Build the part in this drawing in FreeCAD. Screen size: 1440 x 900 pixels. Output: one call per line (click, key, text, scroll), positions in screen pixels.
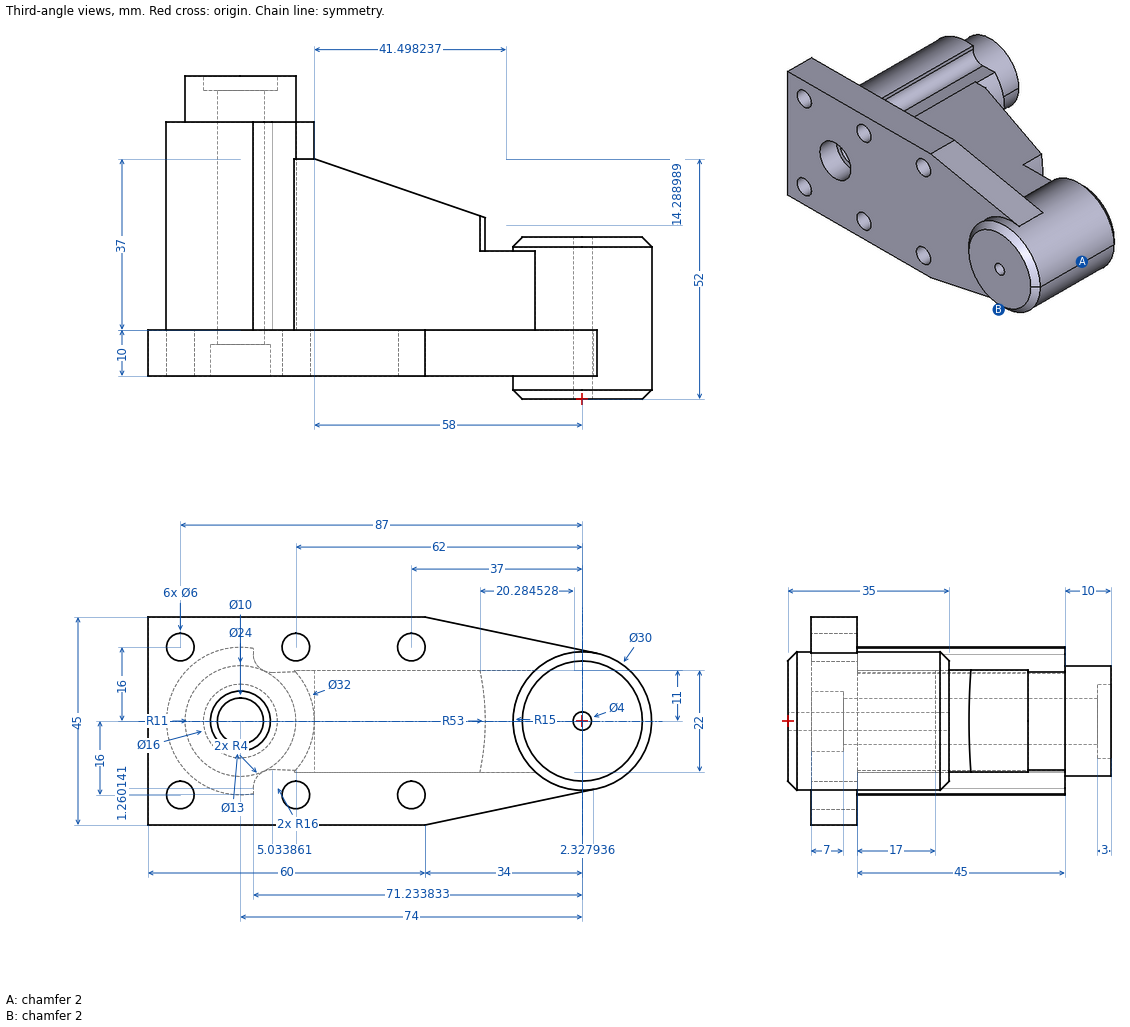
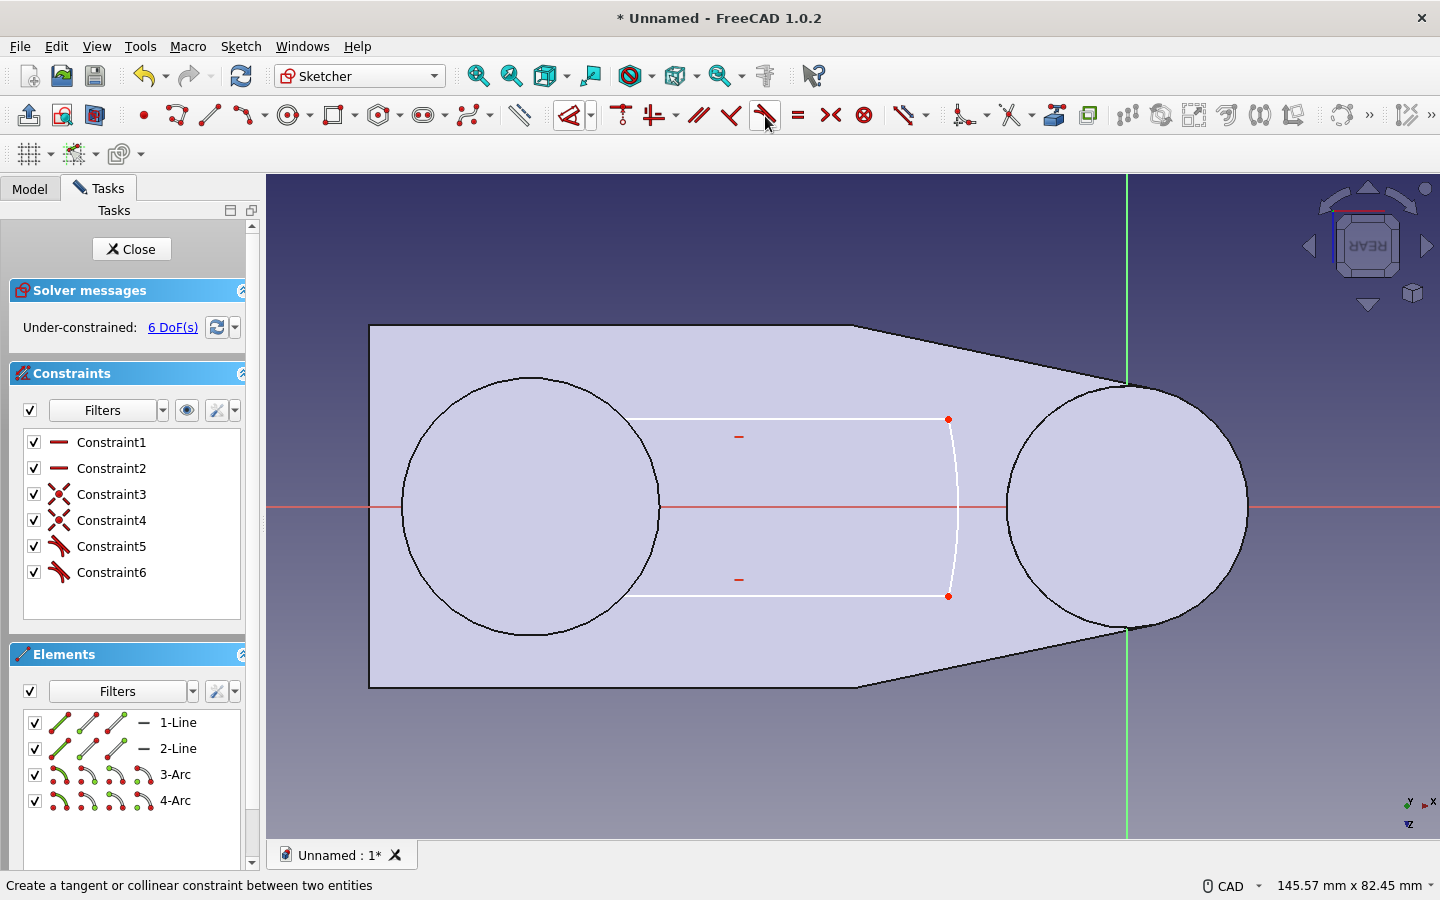
click(459, 456)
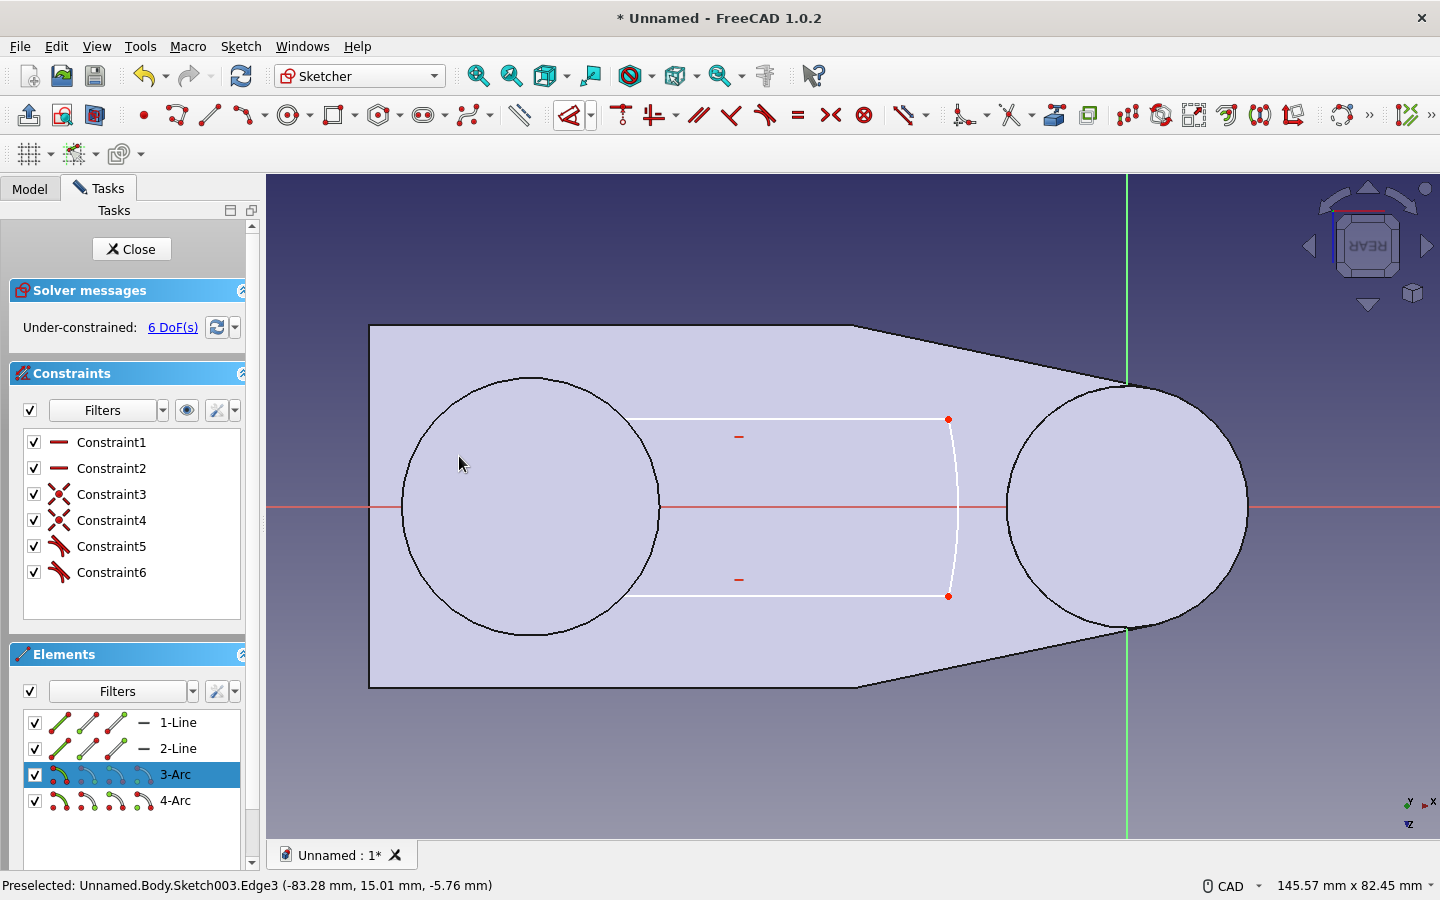
click(957, 544)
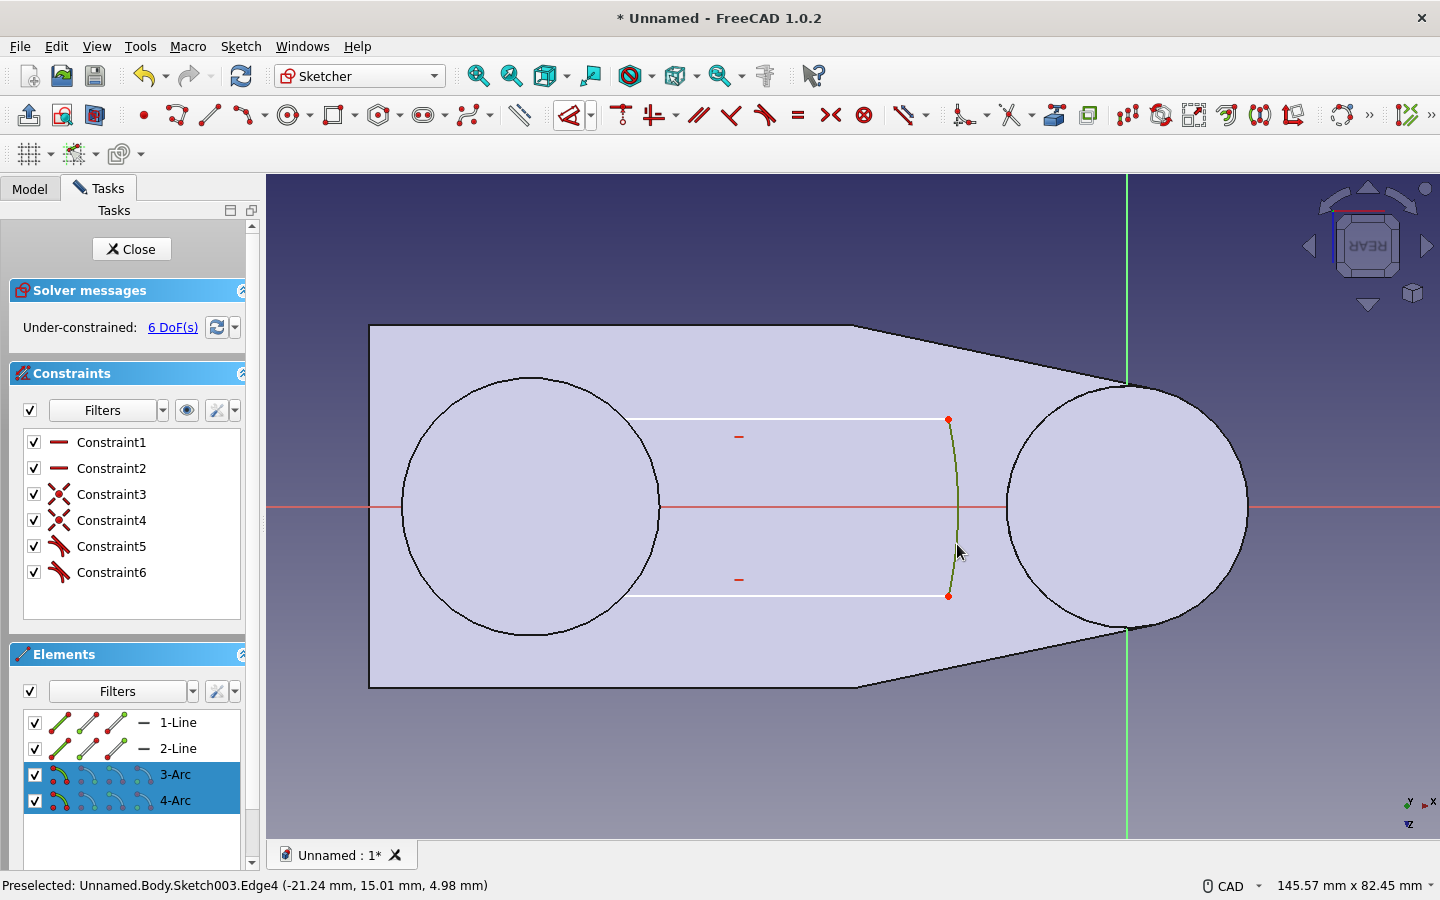
click(621, 116)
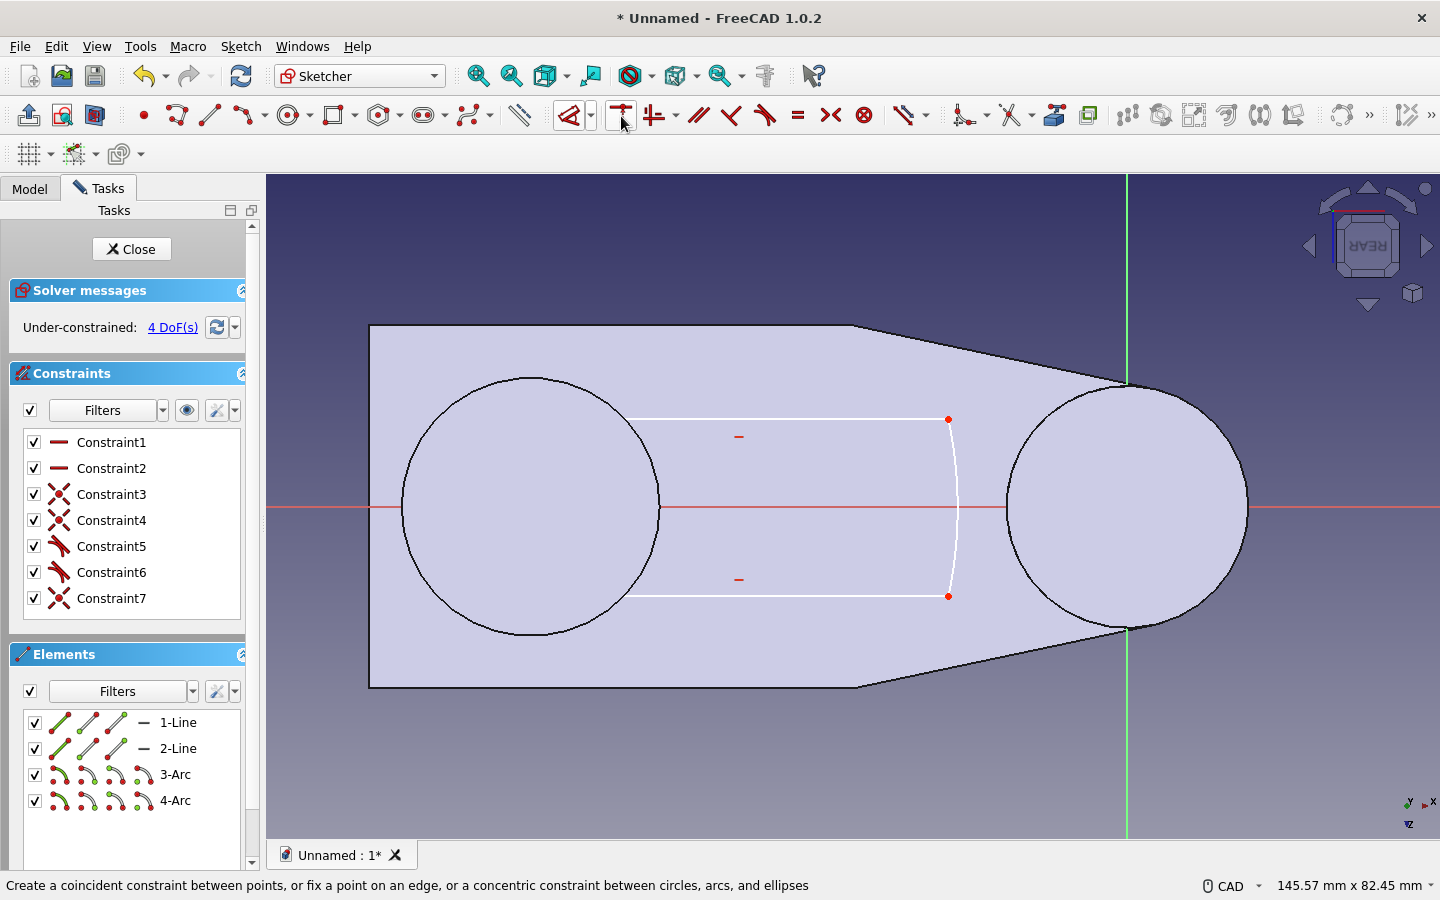
click(531, 508)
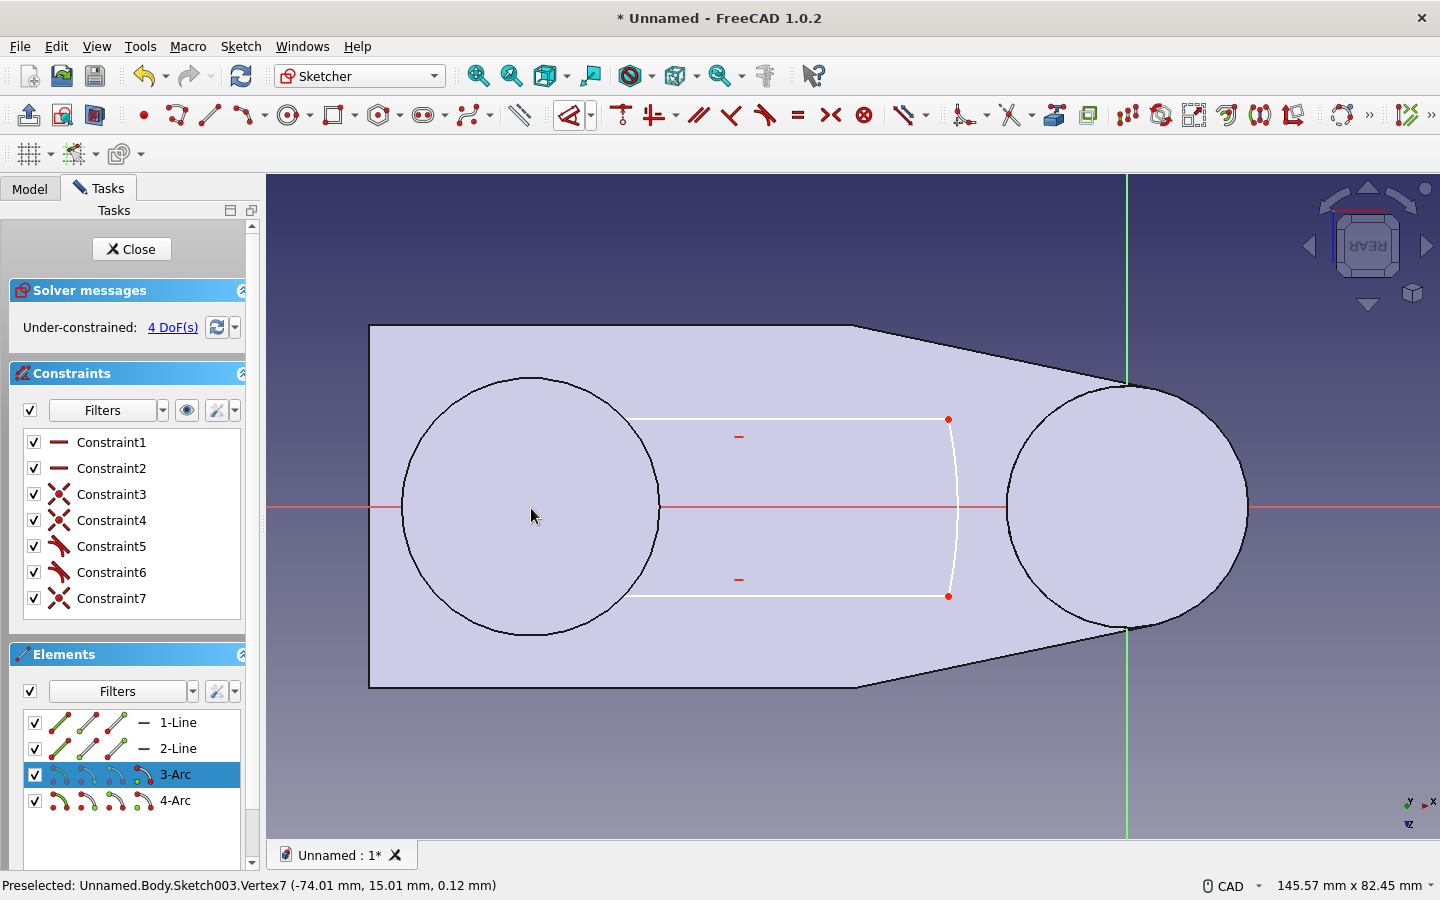
click(364, 507)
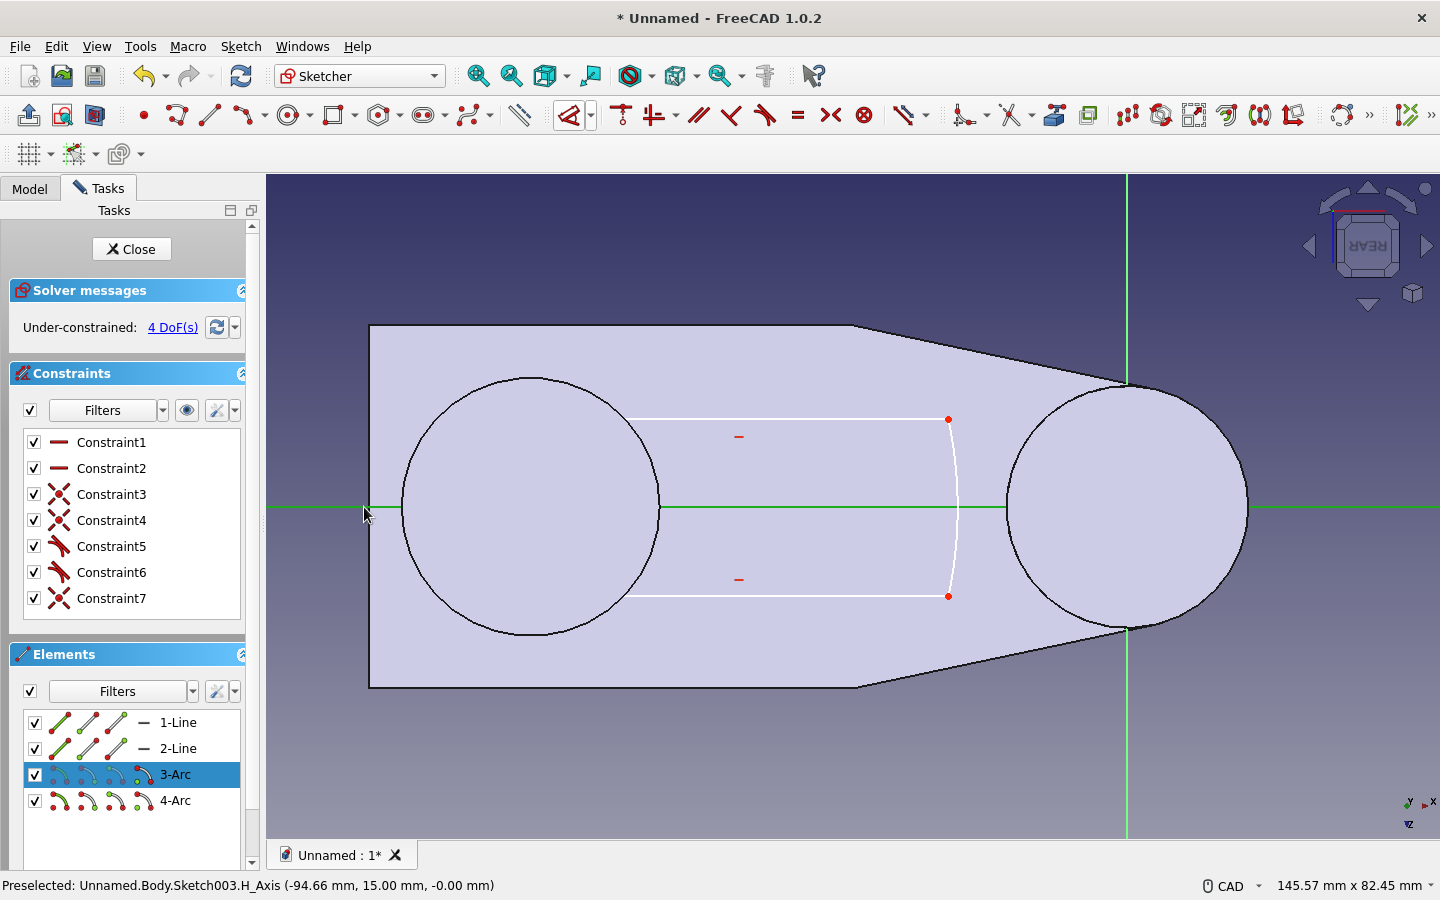
click(621, 116)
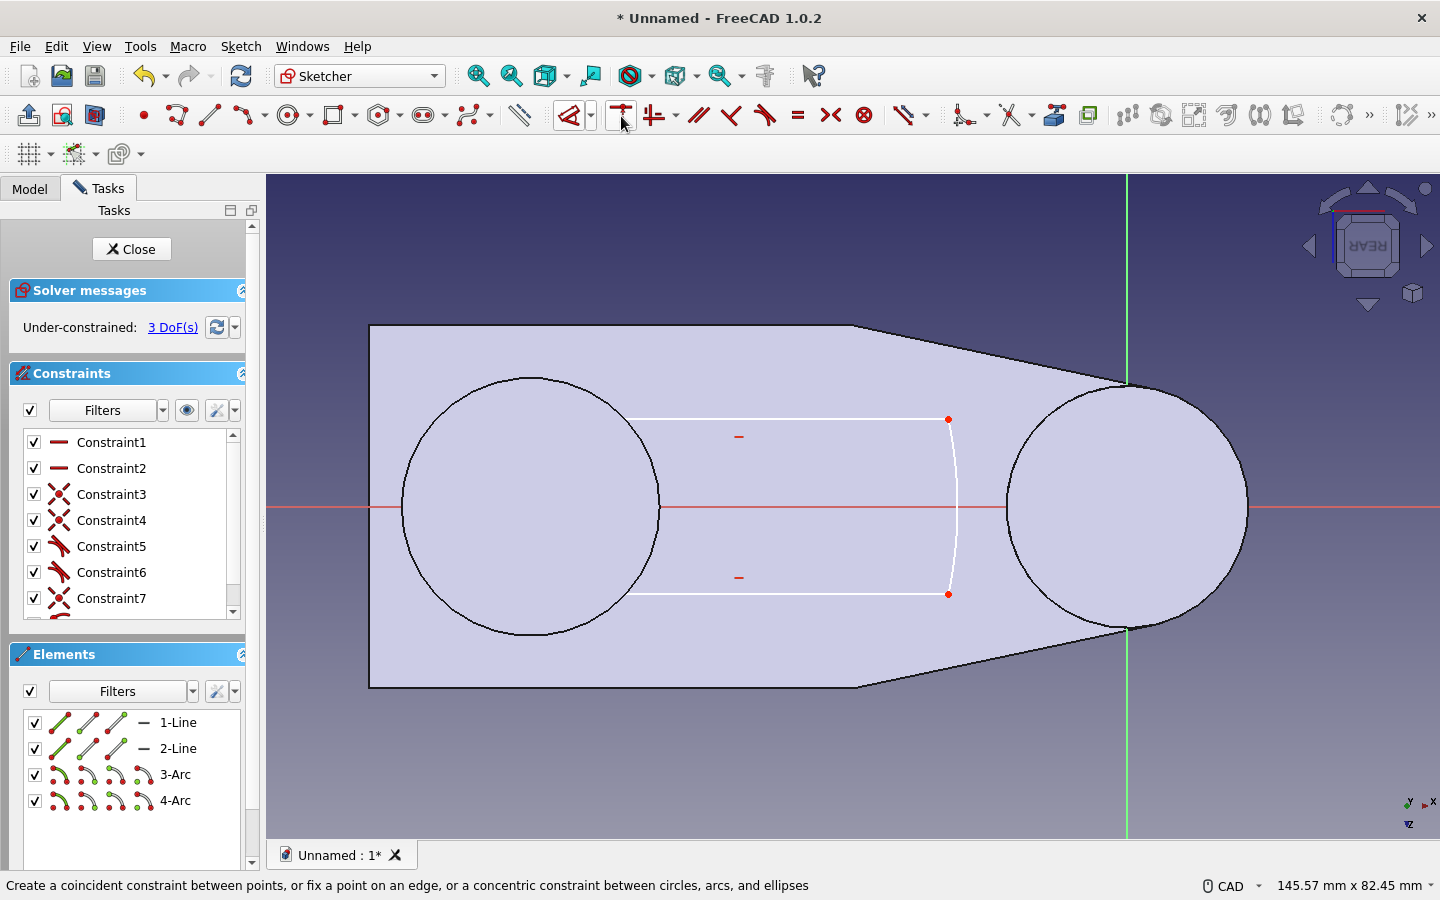
click(460, 456)